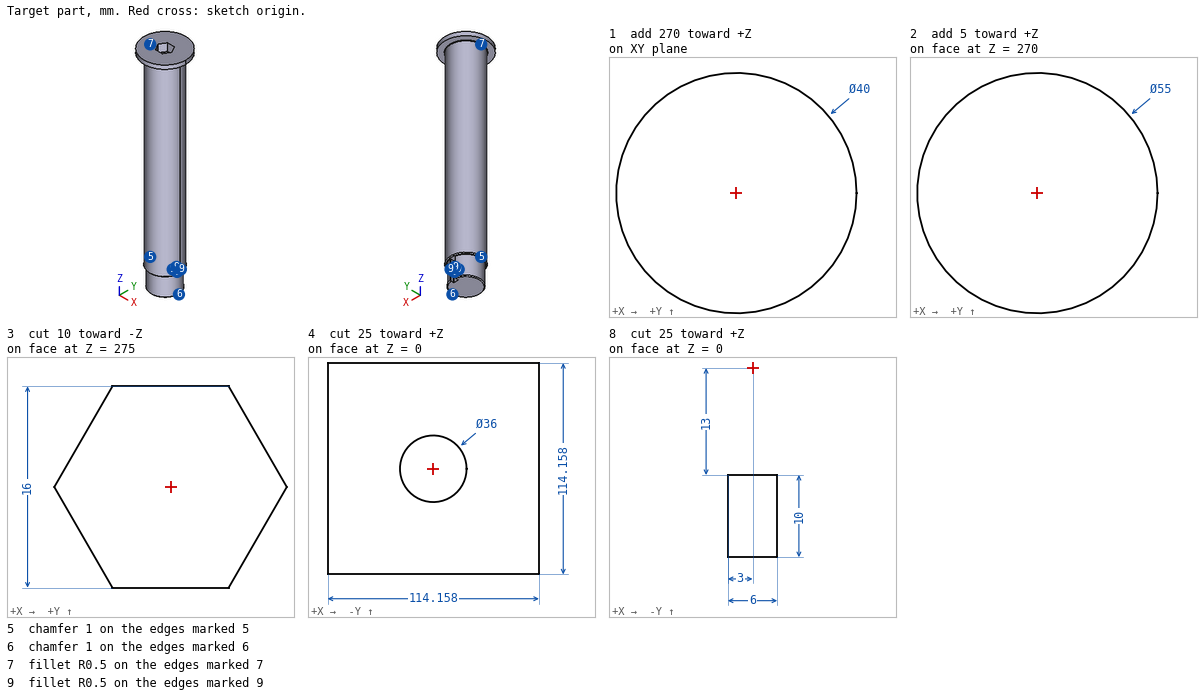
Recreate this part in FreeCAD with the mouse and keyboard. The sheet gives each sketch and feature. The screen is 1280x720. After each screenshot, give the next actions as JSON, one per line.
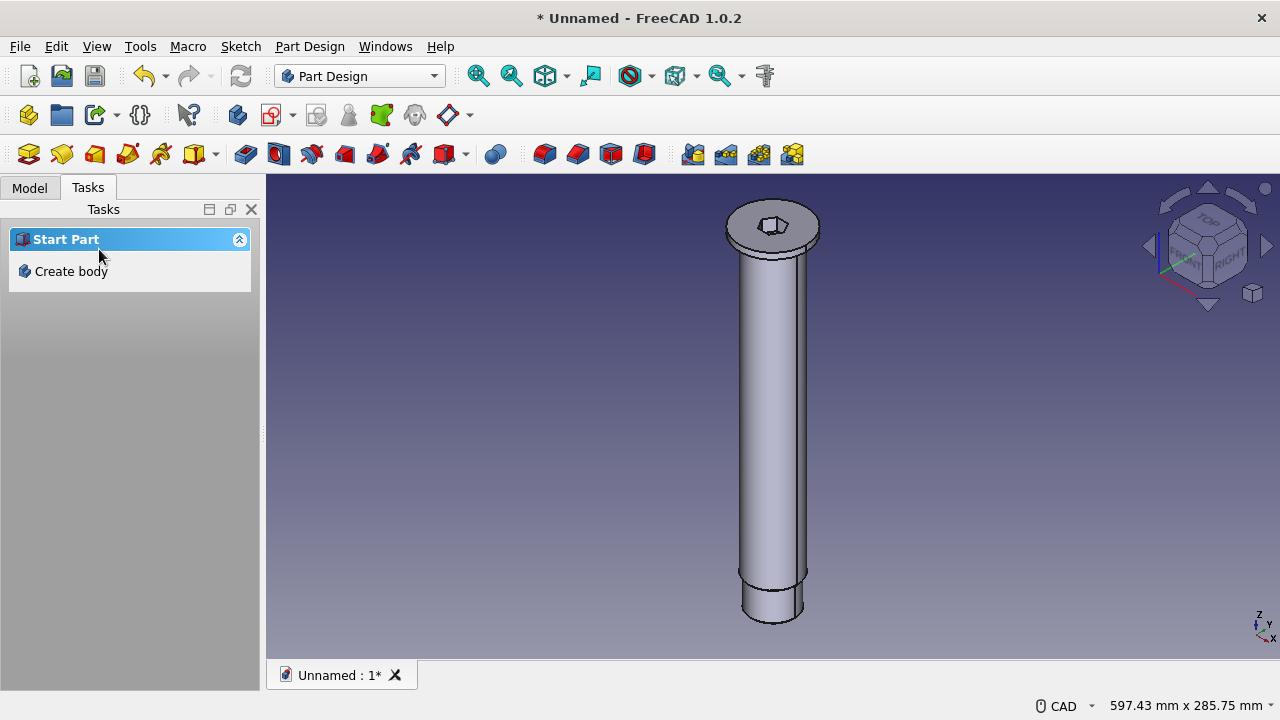
{"action": "key", "text": "2"}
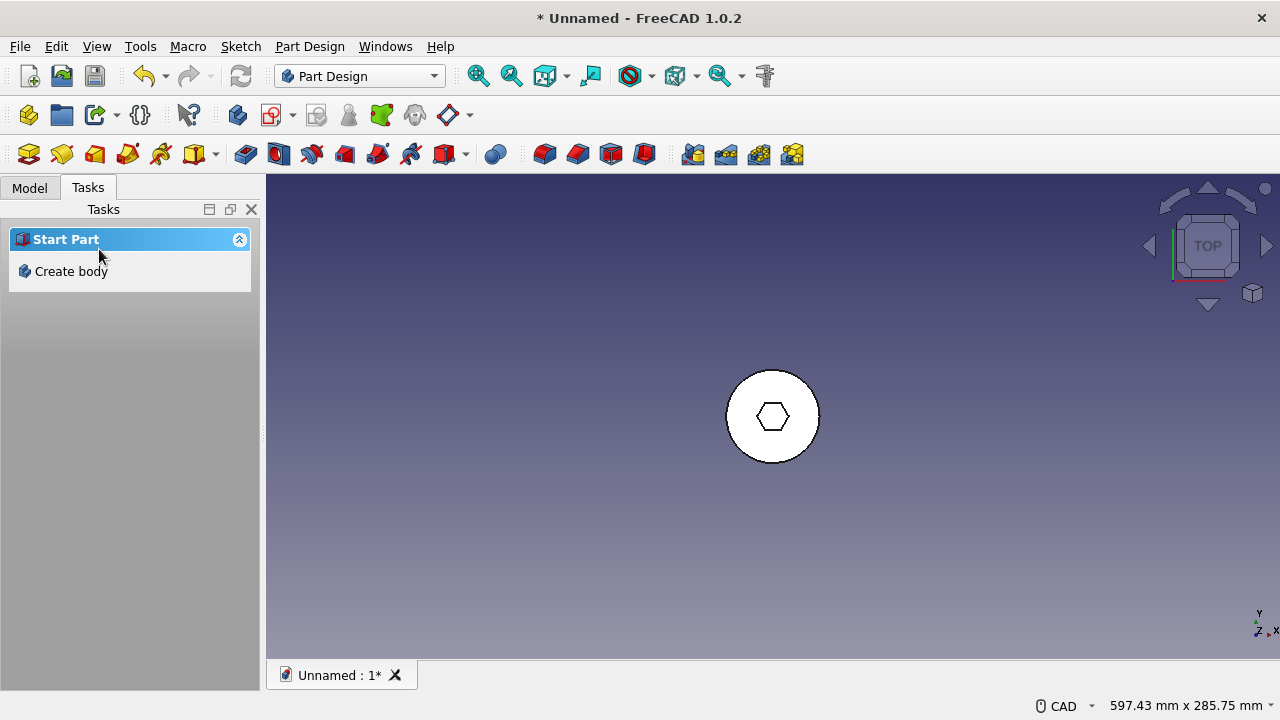
{"action": "left_click", "coordinate": [479, 76]}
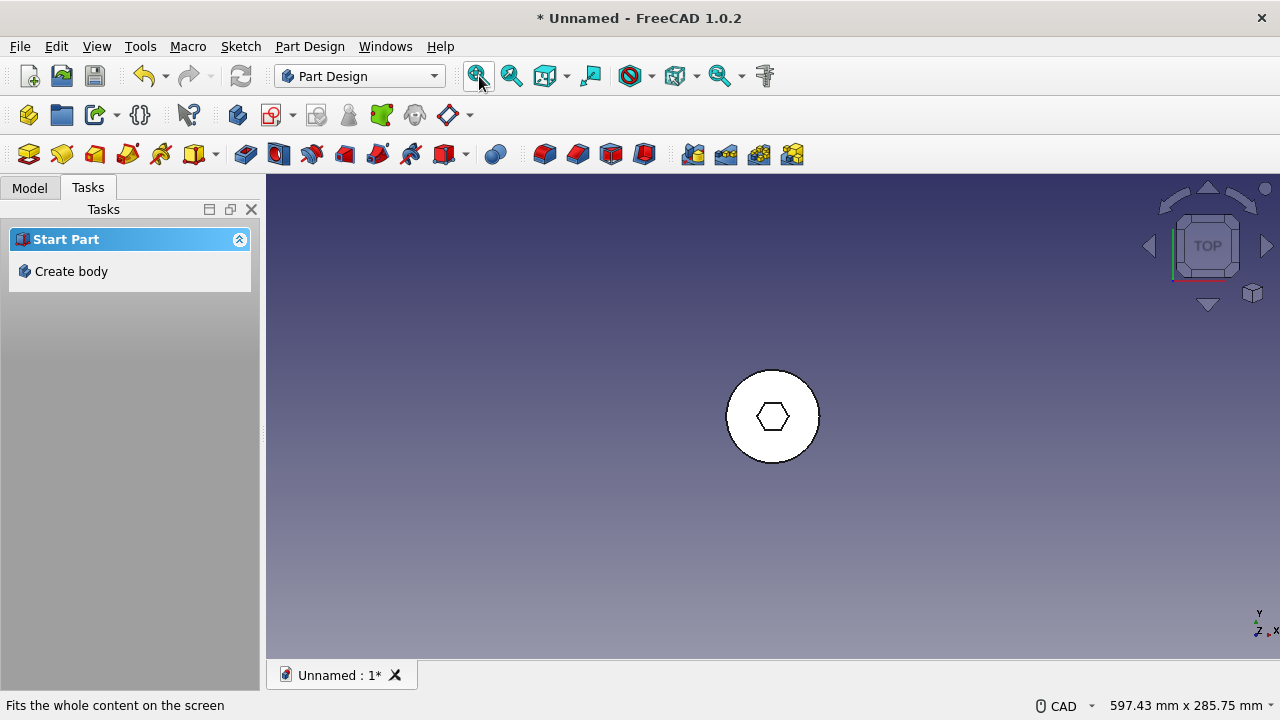
{"action": "key", "text": "0"}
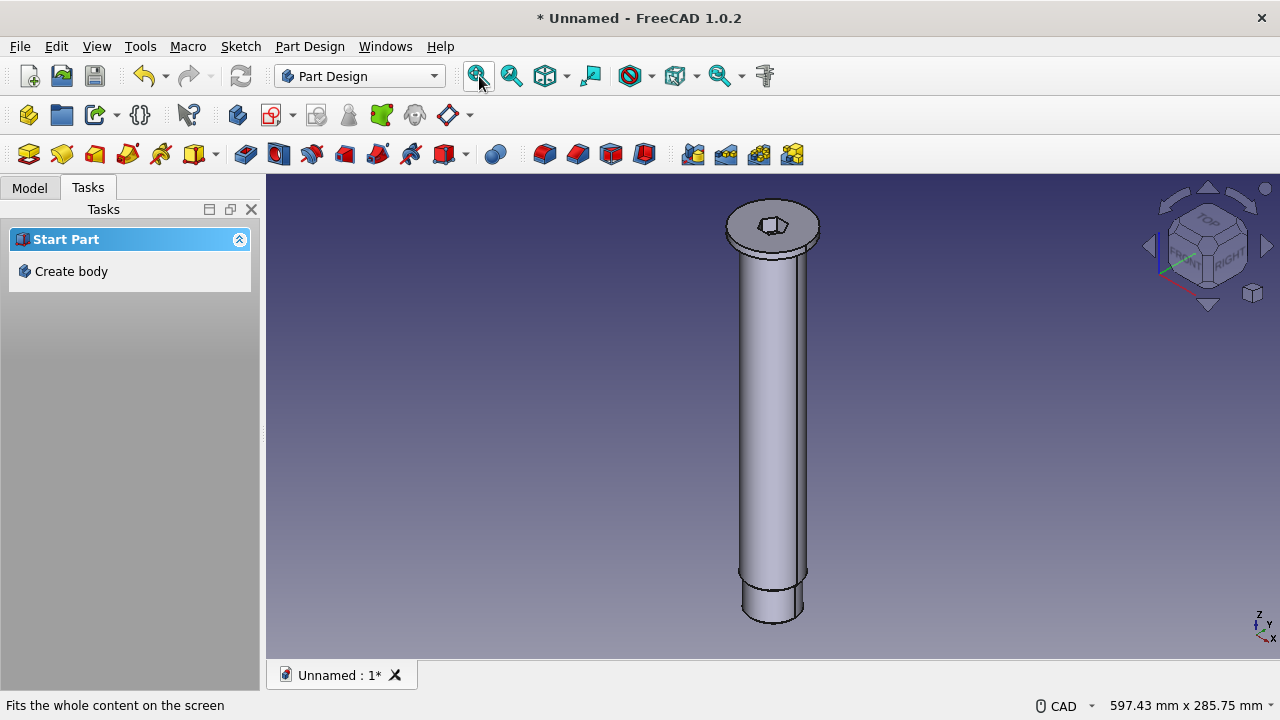
{"action": "key", "text": "1"}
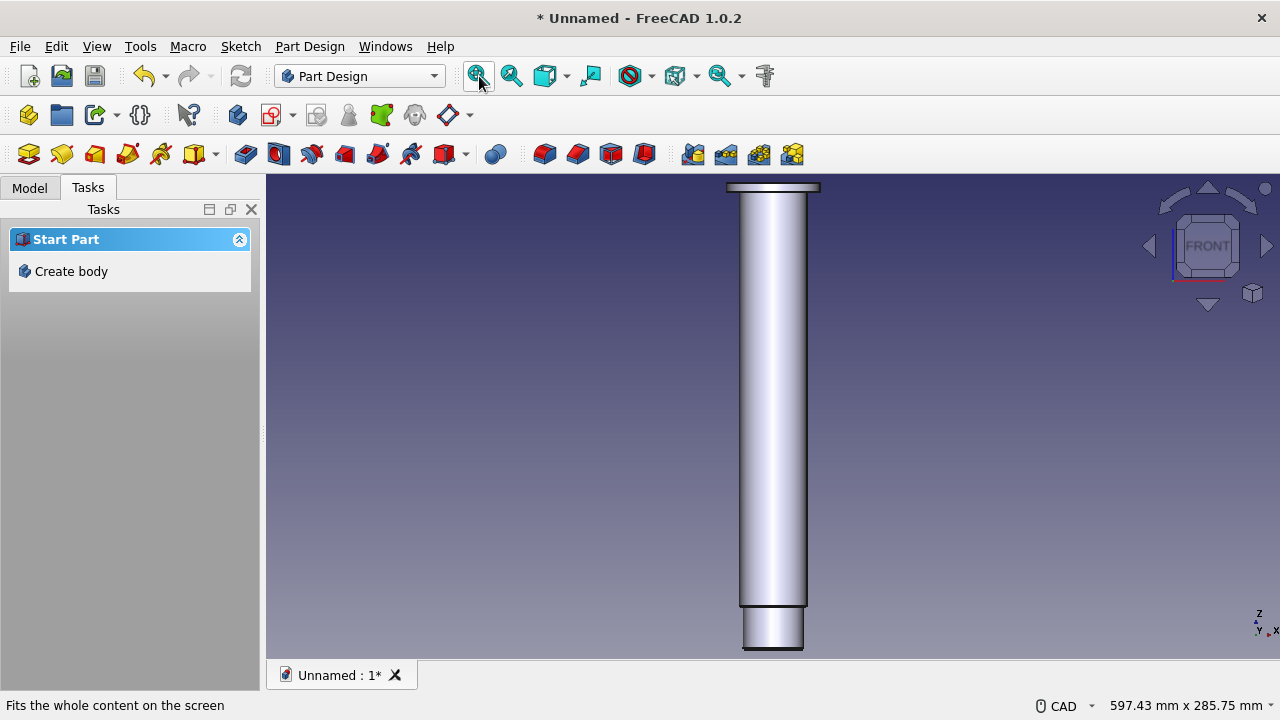
{"action": "key", "text": "3"}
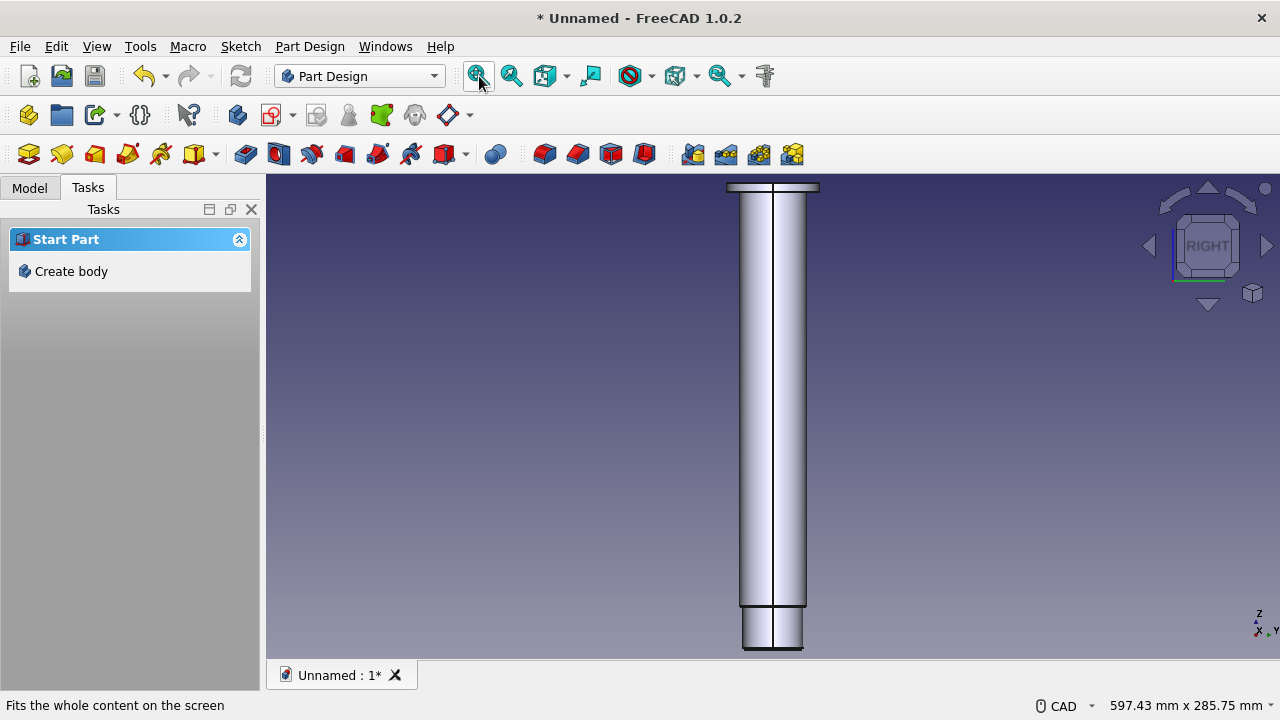
{"action": "key", "text": "5"}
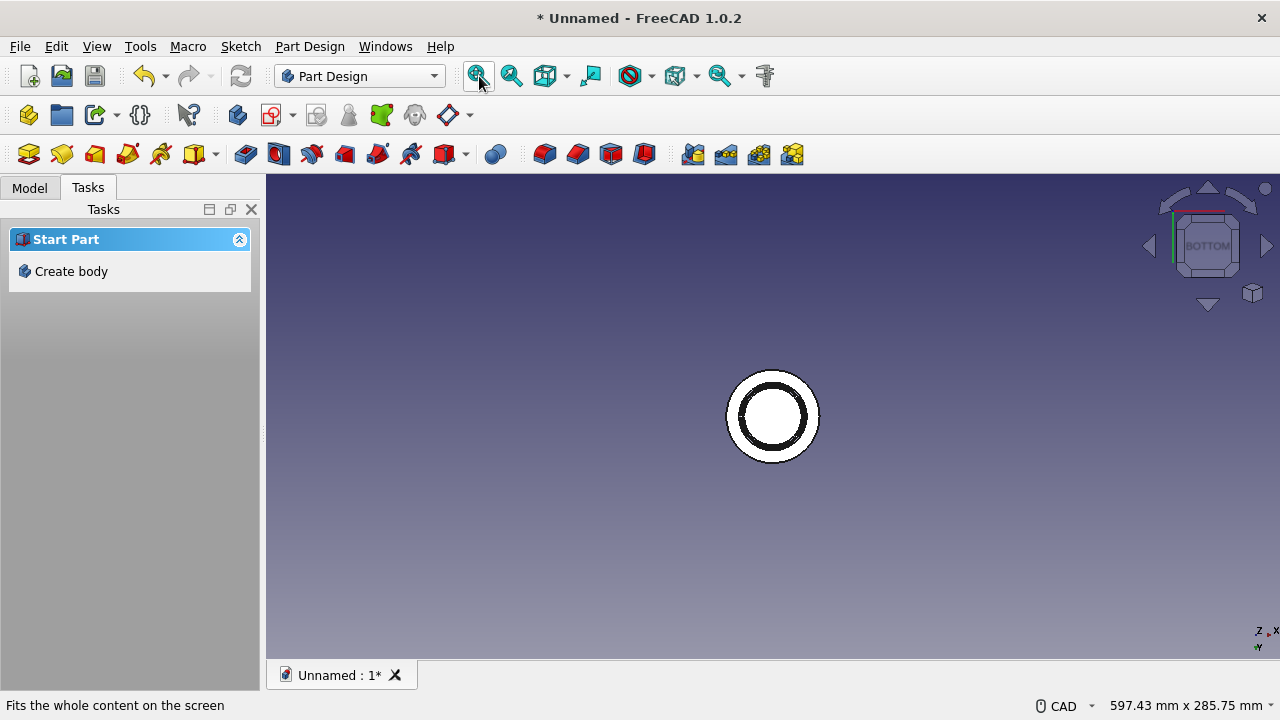
{"action": "left_click", "coordinate": [479, 76]}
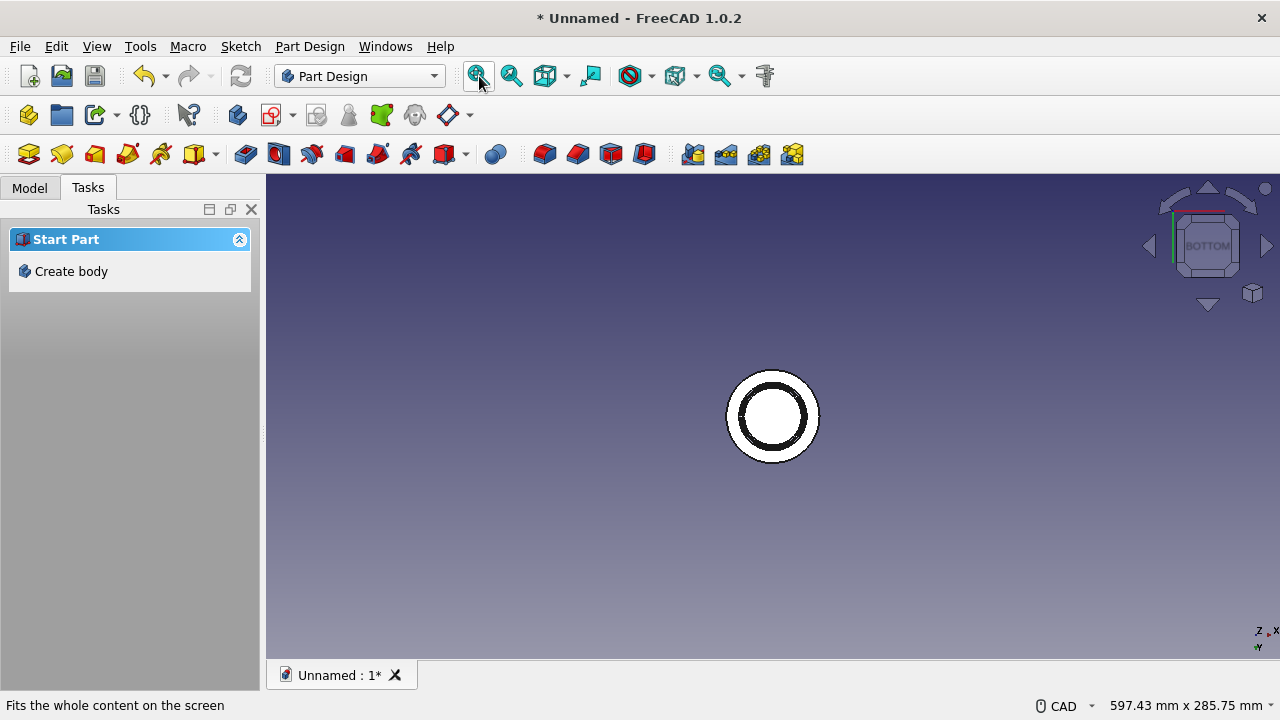
{"action": "key", "text": "4"}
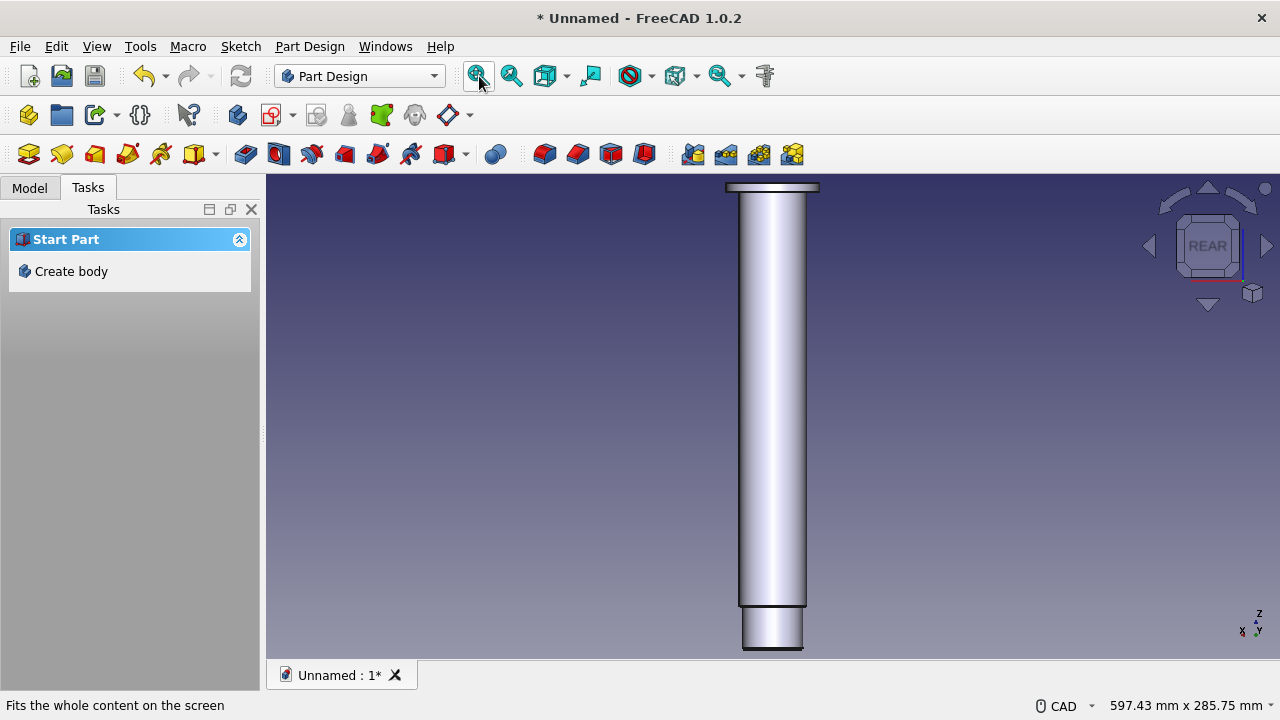
{"action": "key", "text": "6"}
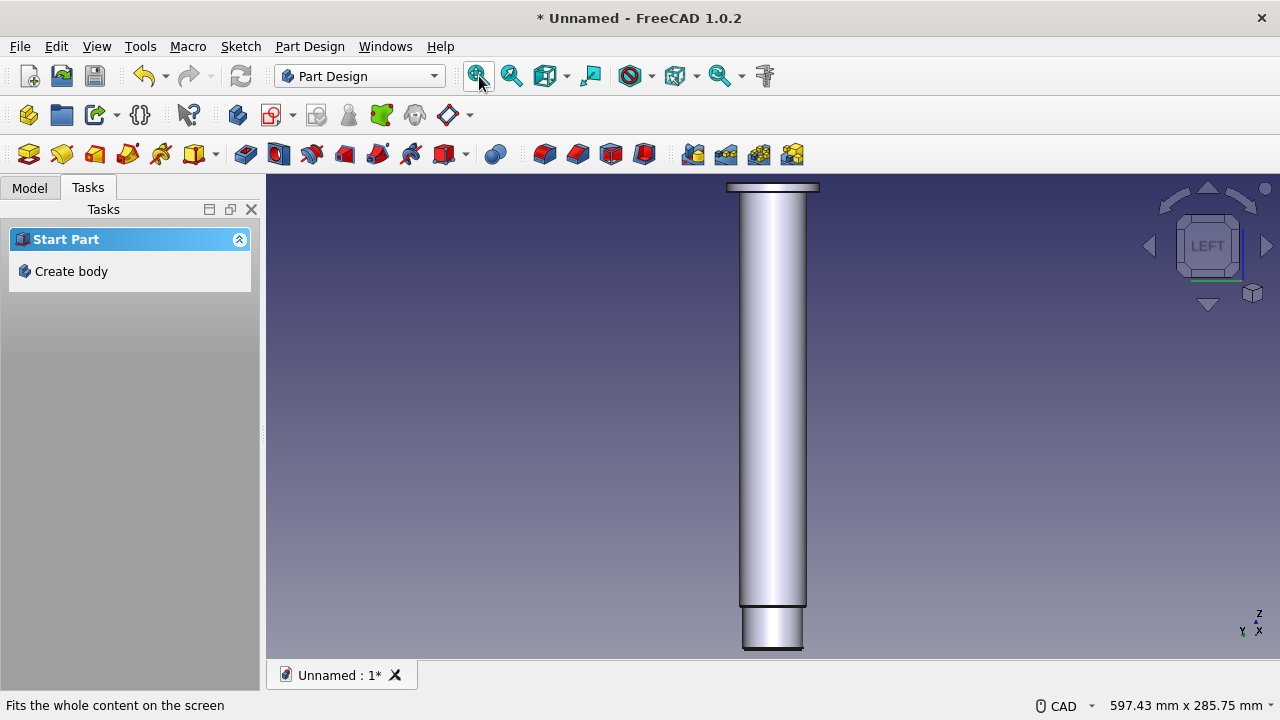
{"action": "key", "text": "v 3"}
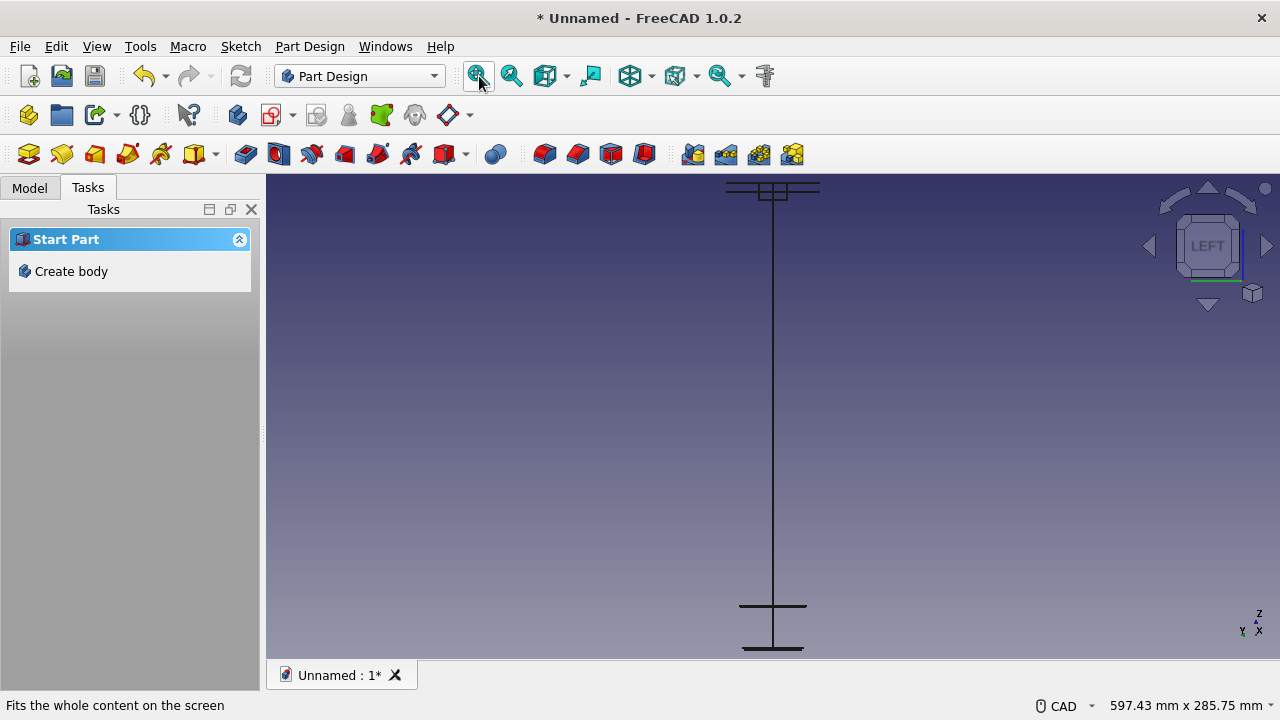
{"action": "key", "text": "0"}